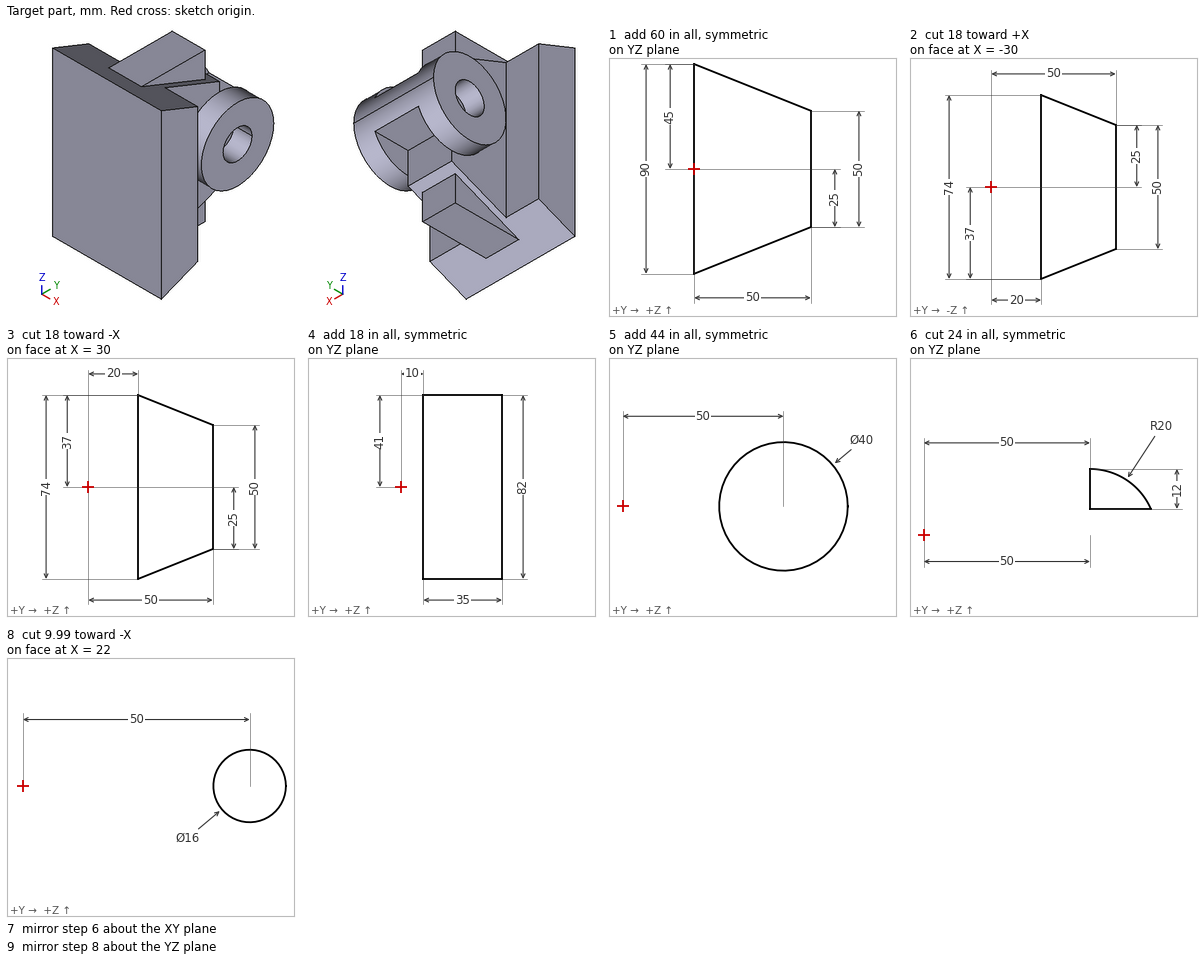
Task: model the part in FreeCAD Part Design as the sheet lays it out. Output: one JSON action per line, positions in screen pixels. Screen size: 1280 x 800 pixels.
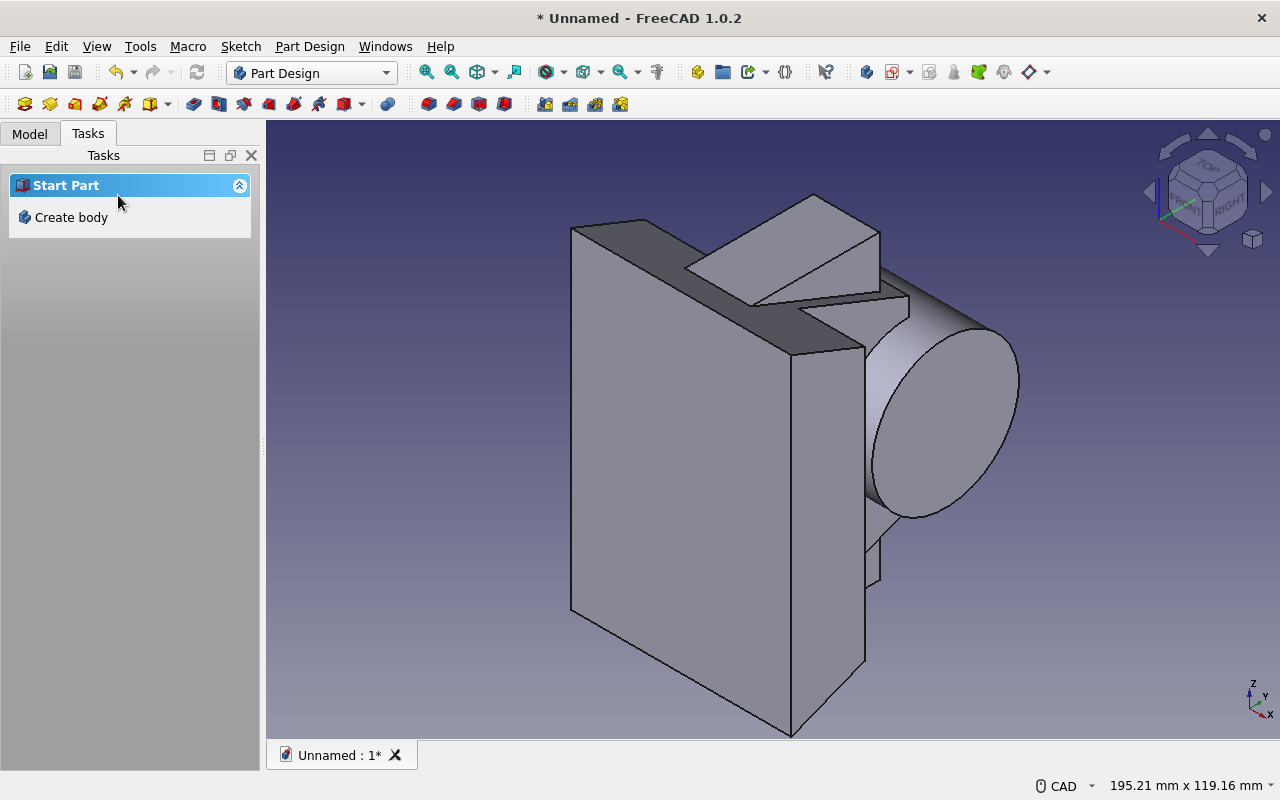
{"action": "left_click", "coordinate": [427, 72]}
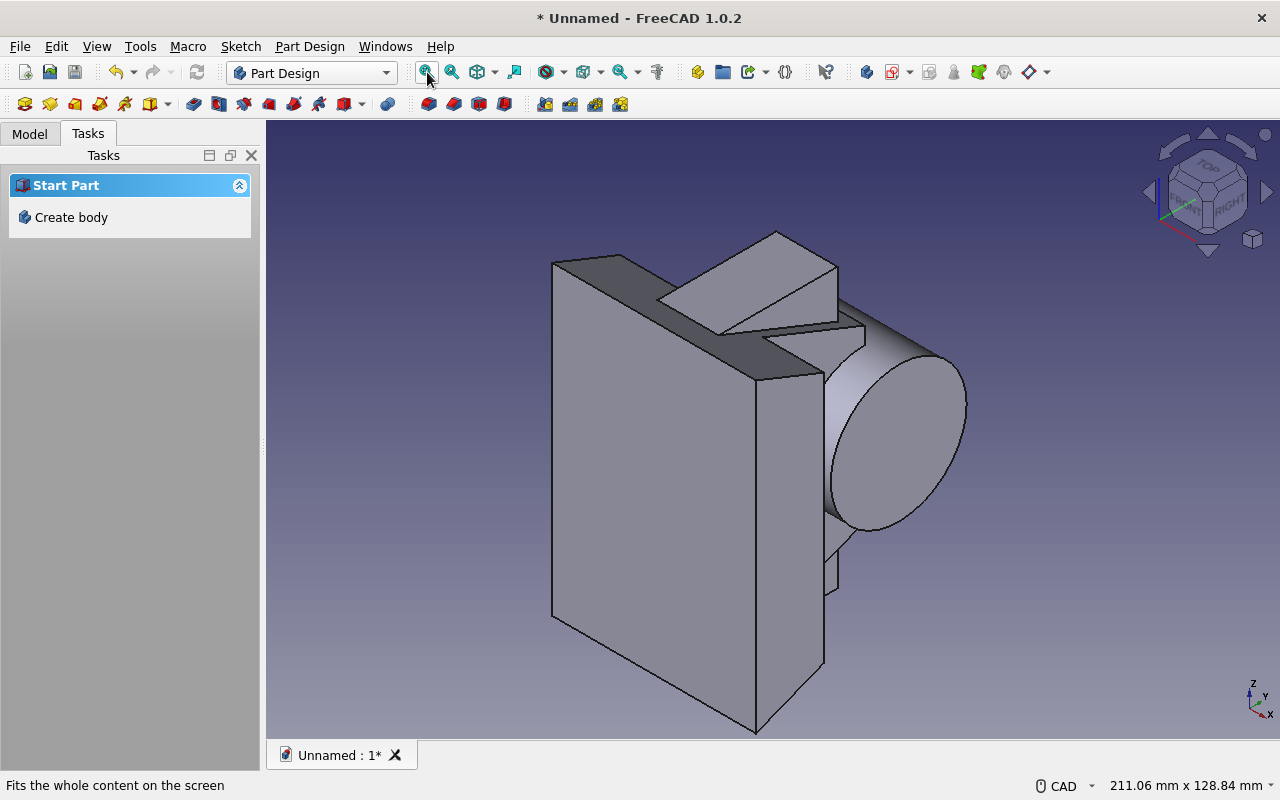
{"action": "left_click", "coordinate": [892, 72]}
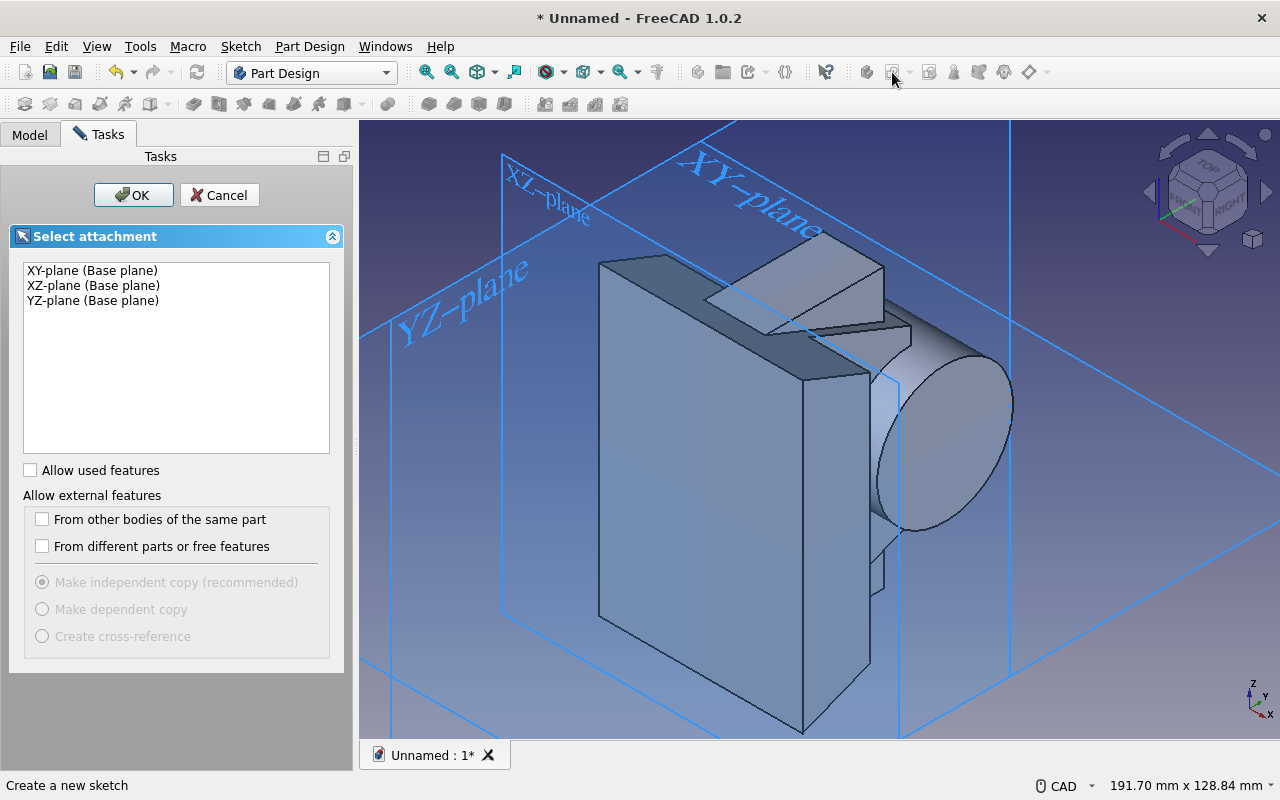
{"action": "left_click", "coordinate": [84, 300]}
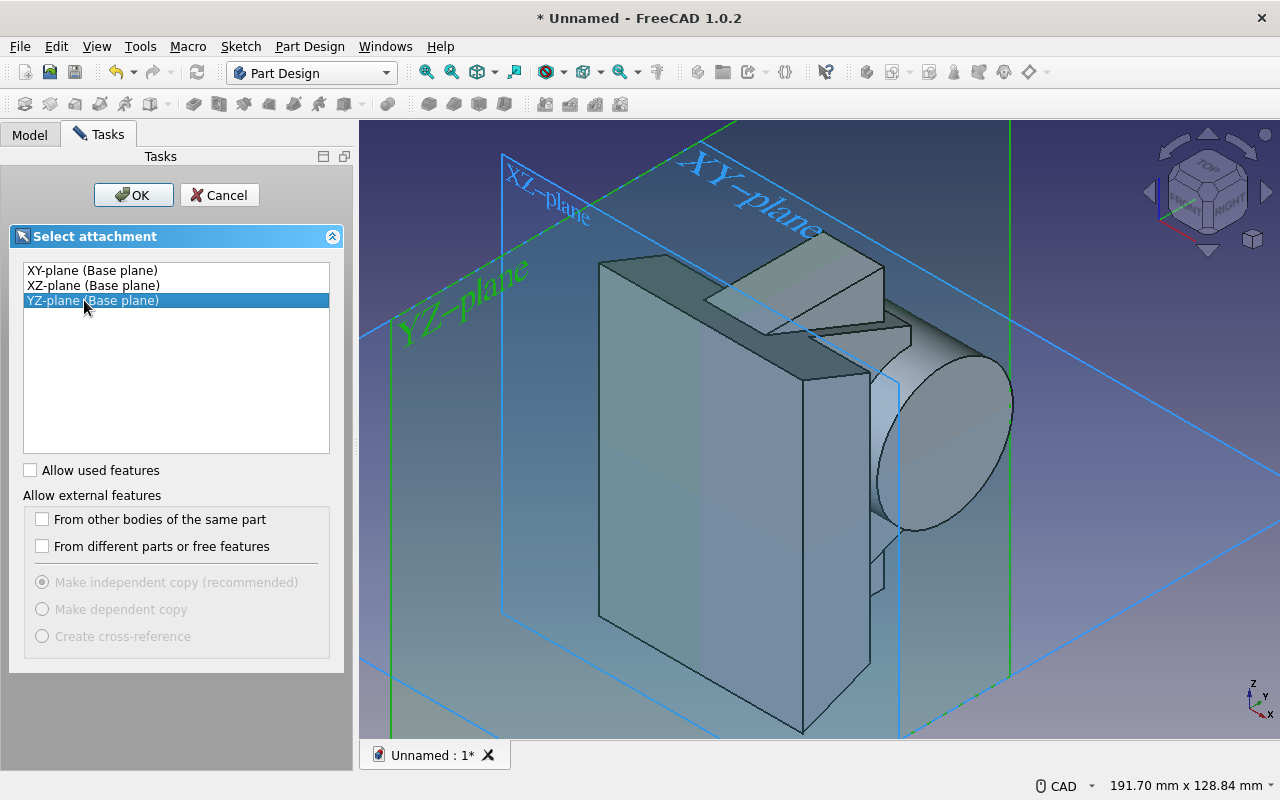
{"action": "left_click", "coordinate": [134, 195]}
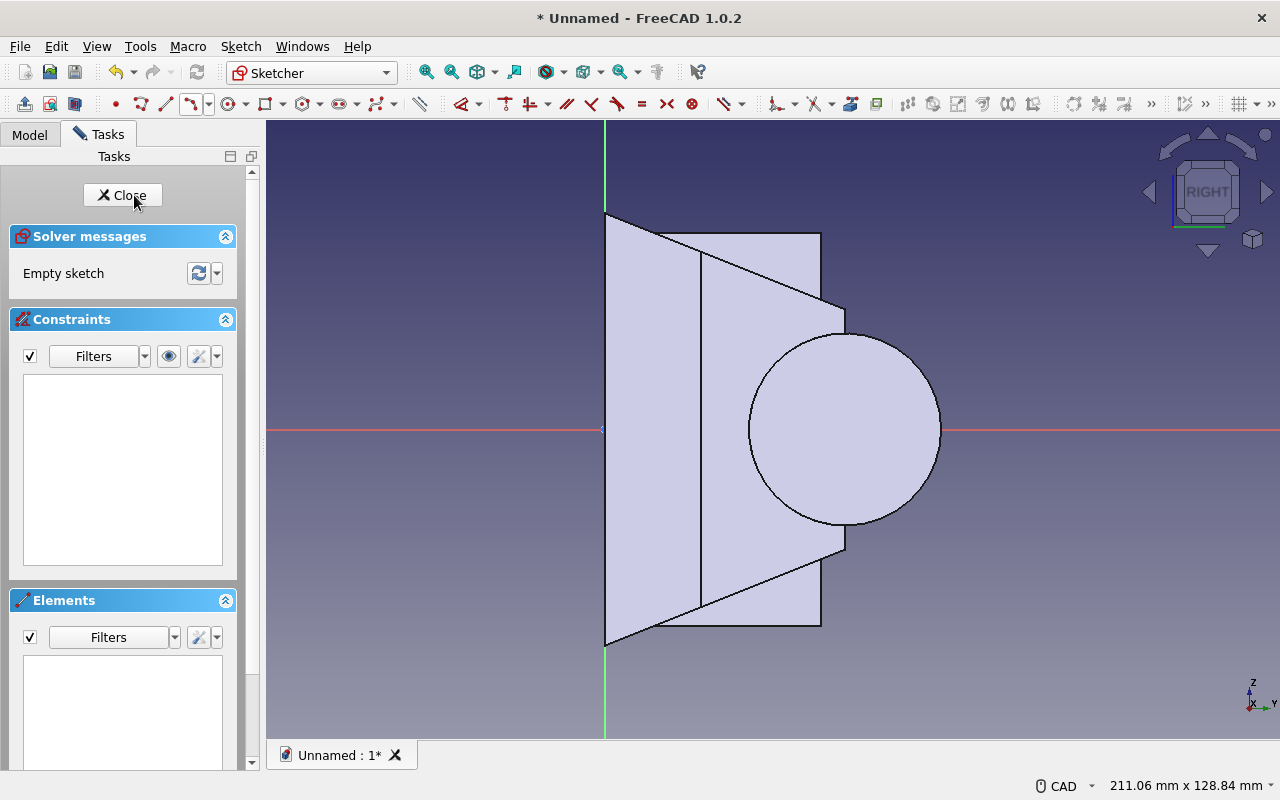
{"action": "left_click", "coordinate": [75, 104]}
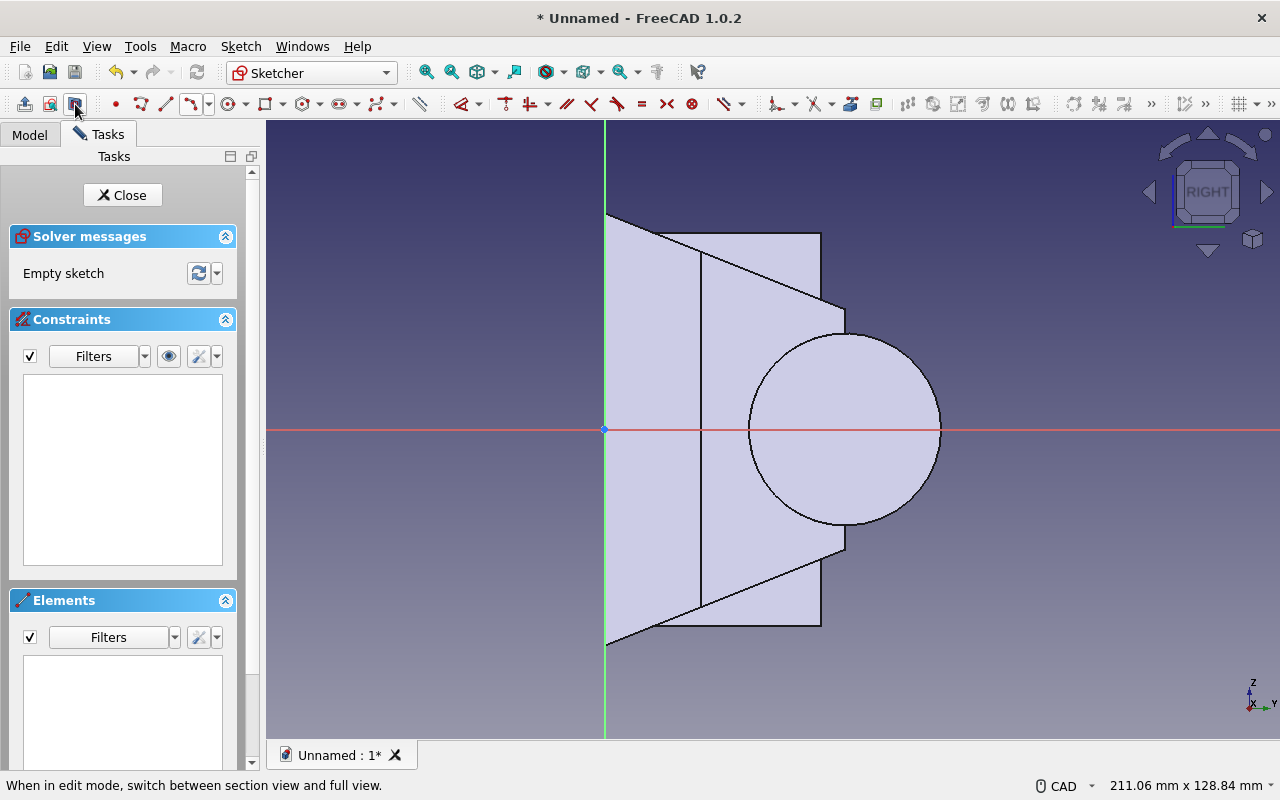
{"action": "scroll", "coordinate": [926, 349], "scroll_direction": "up", "scroll_amount": 9}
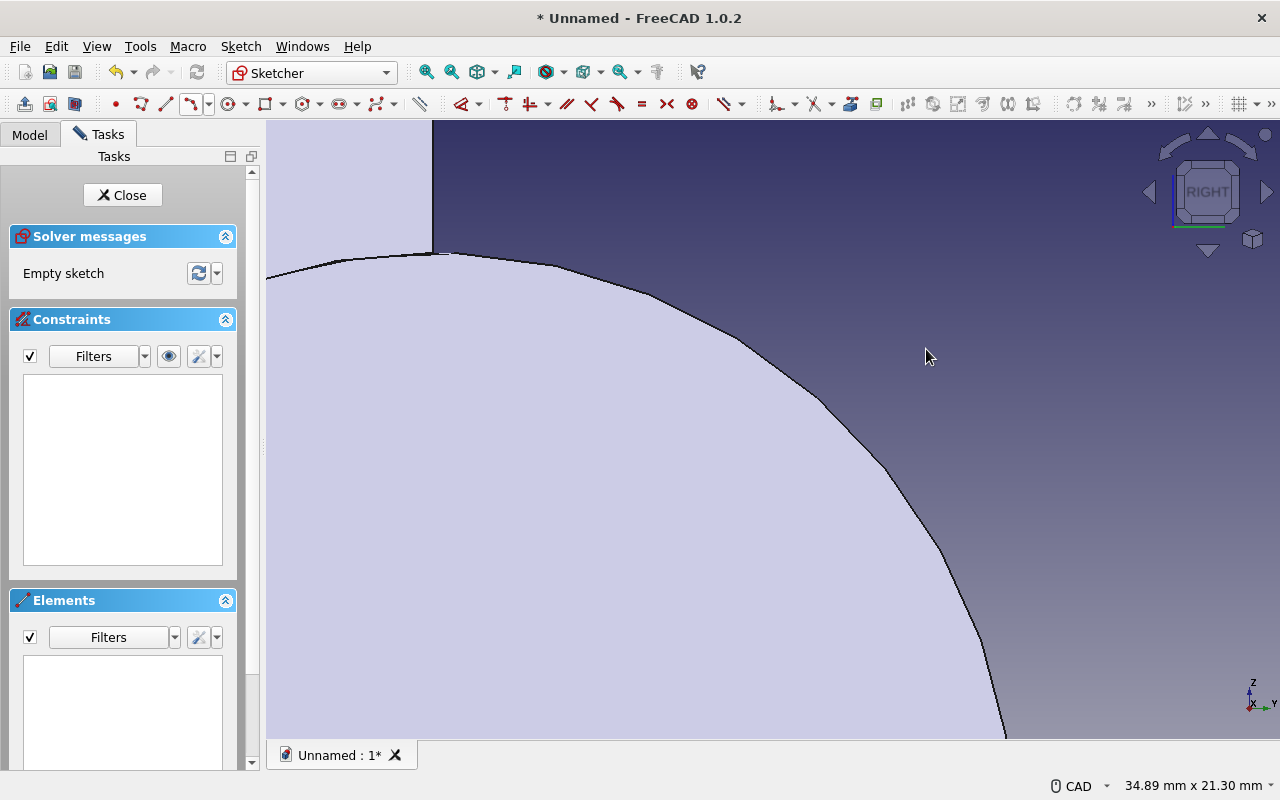
{"action": "left_click", "coordinate": [141, 104]}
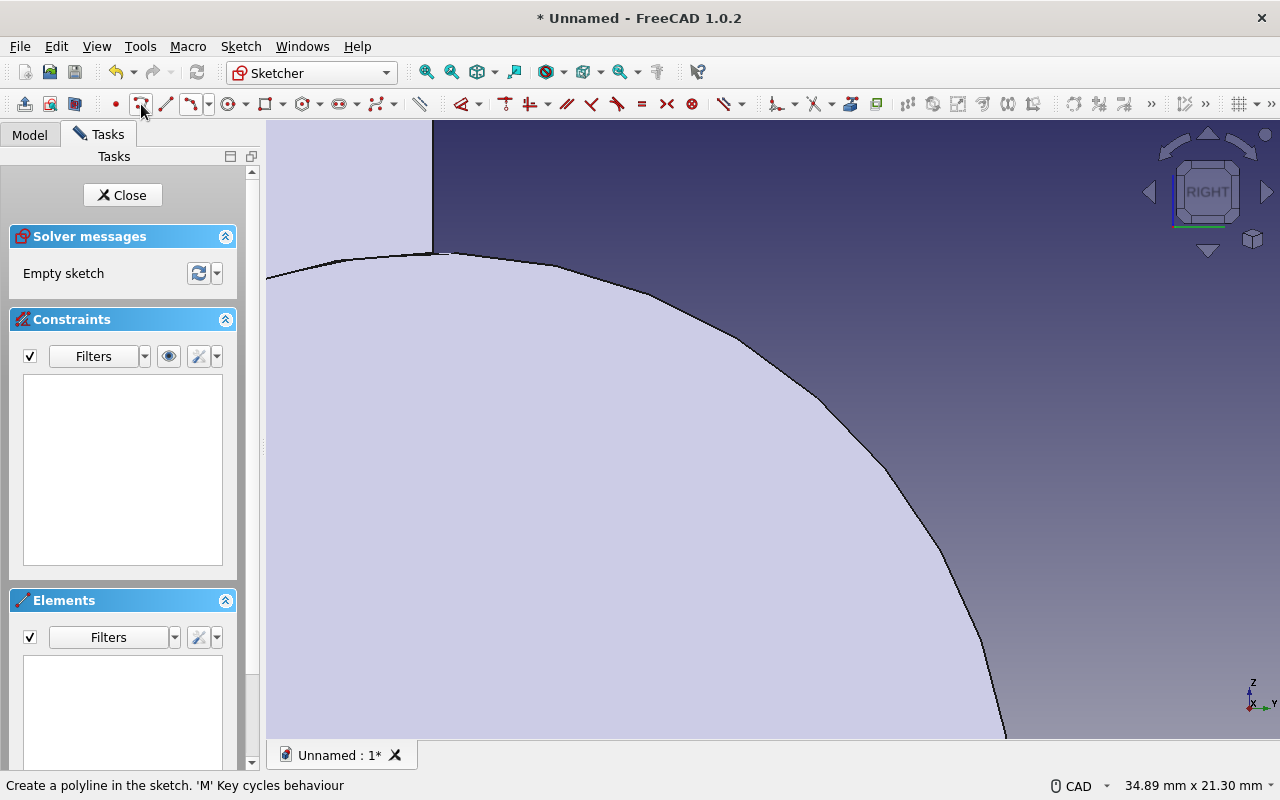
{"action": "left_click", "coordinate": [433, 253]}
{"action": "left_click", "coordinate": [433, 602]}
{"action": "left_click", "coordinate": [966, 602]}
{"action": "right_click", "coordinate": [966, 602]}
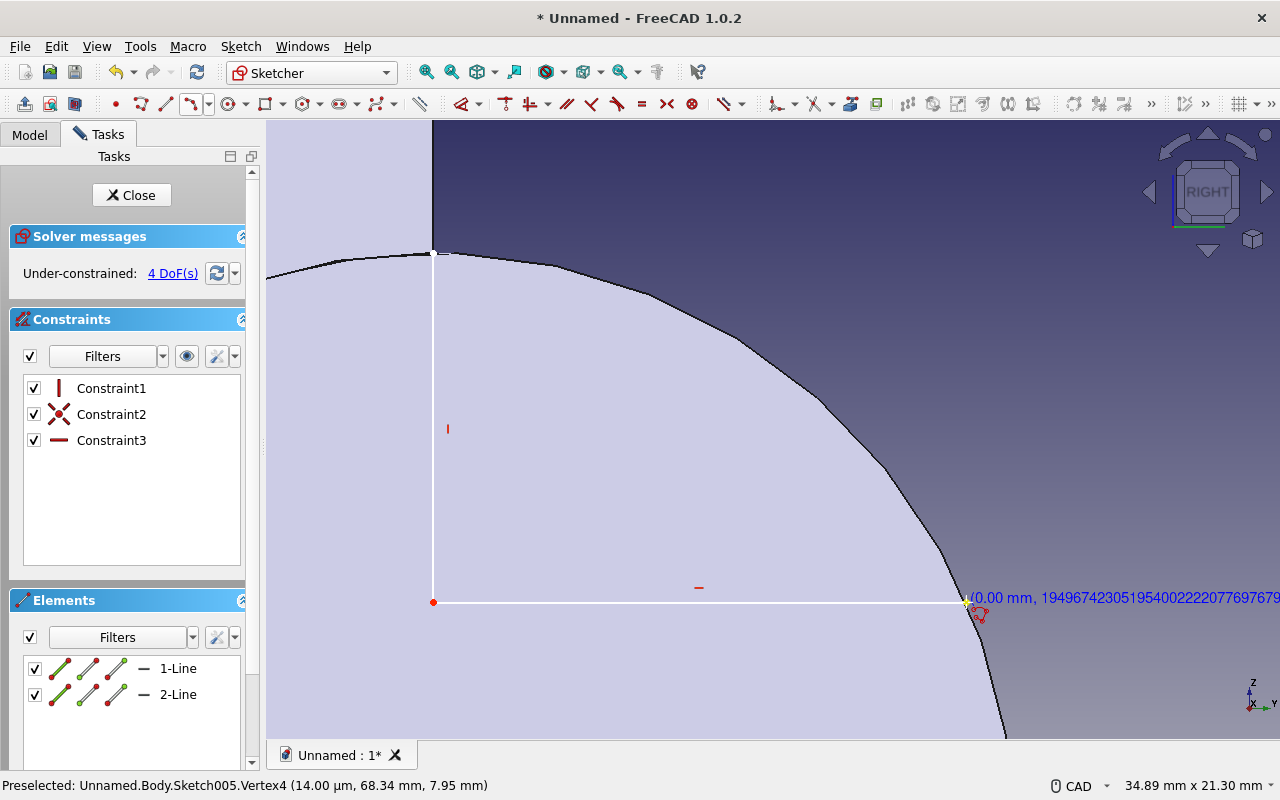
{"action": "key", "text": "g 3 a"}